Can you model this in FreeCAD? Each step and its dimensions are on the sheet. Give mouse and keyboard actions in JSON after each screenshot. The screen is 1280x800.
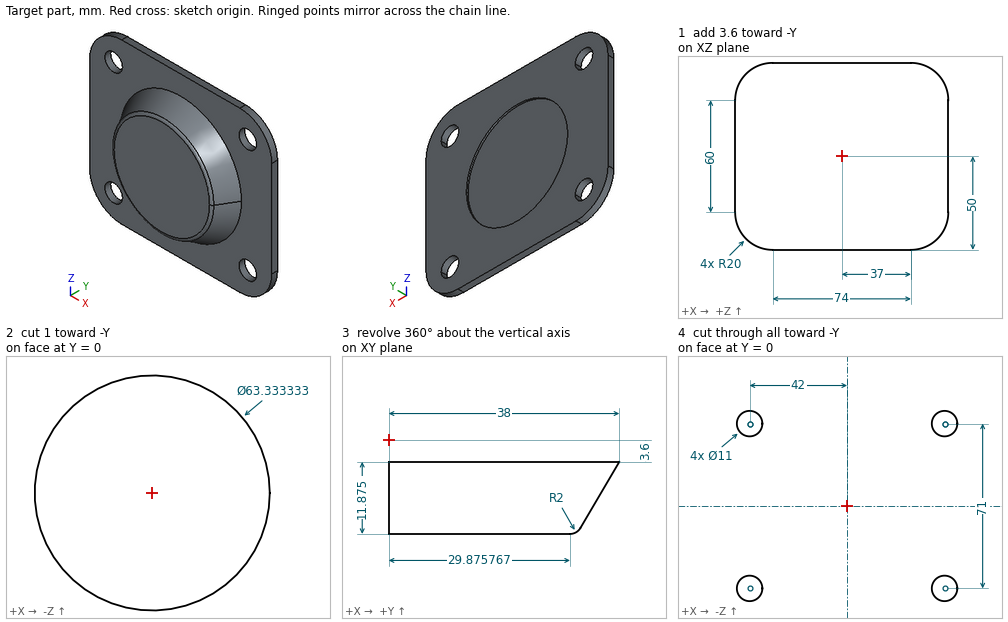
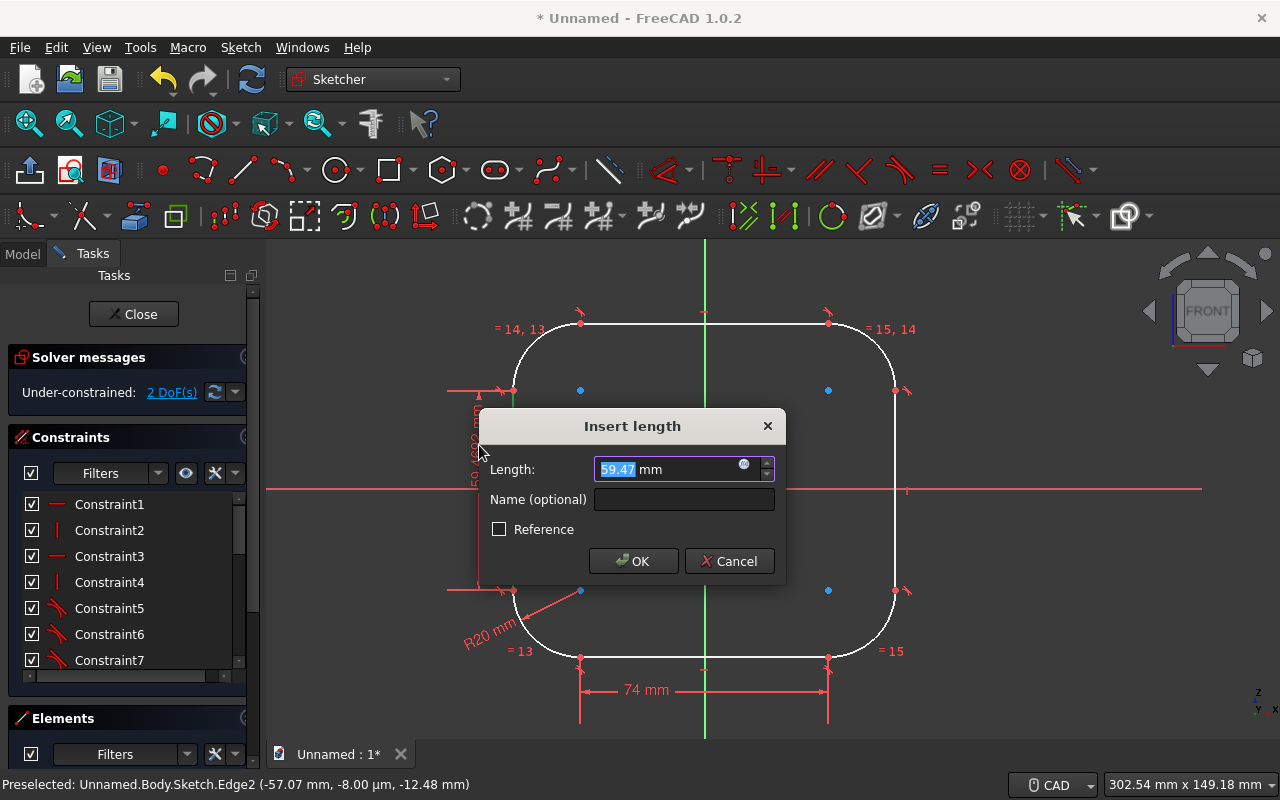
{"action": "type", "text": "60"}
{"action": "key", "text": "Return"}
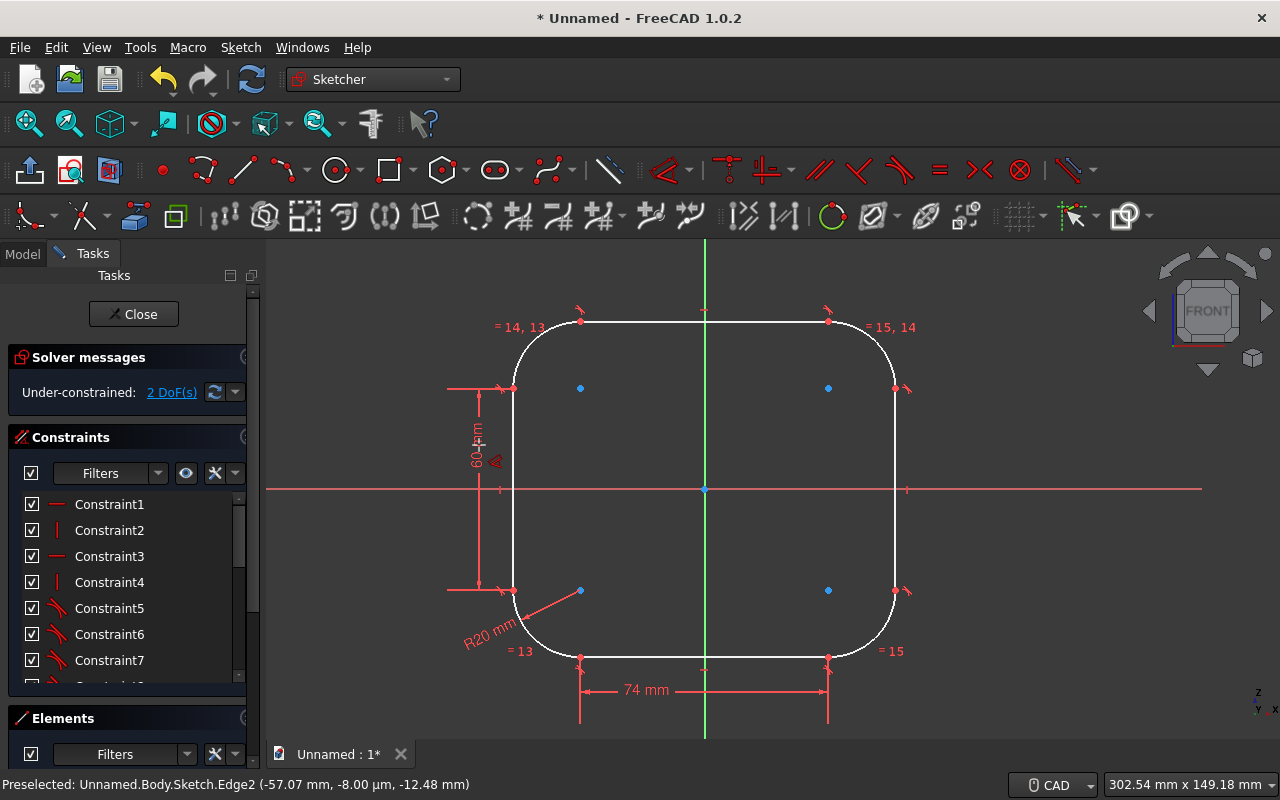
{"action": "left_click", "coordinate": [828, 657]}
{"action": "left_click", "coordinate": [766, 691]}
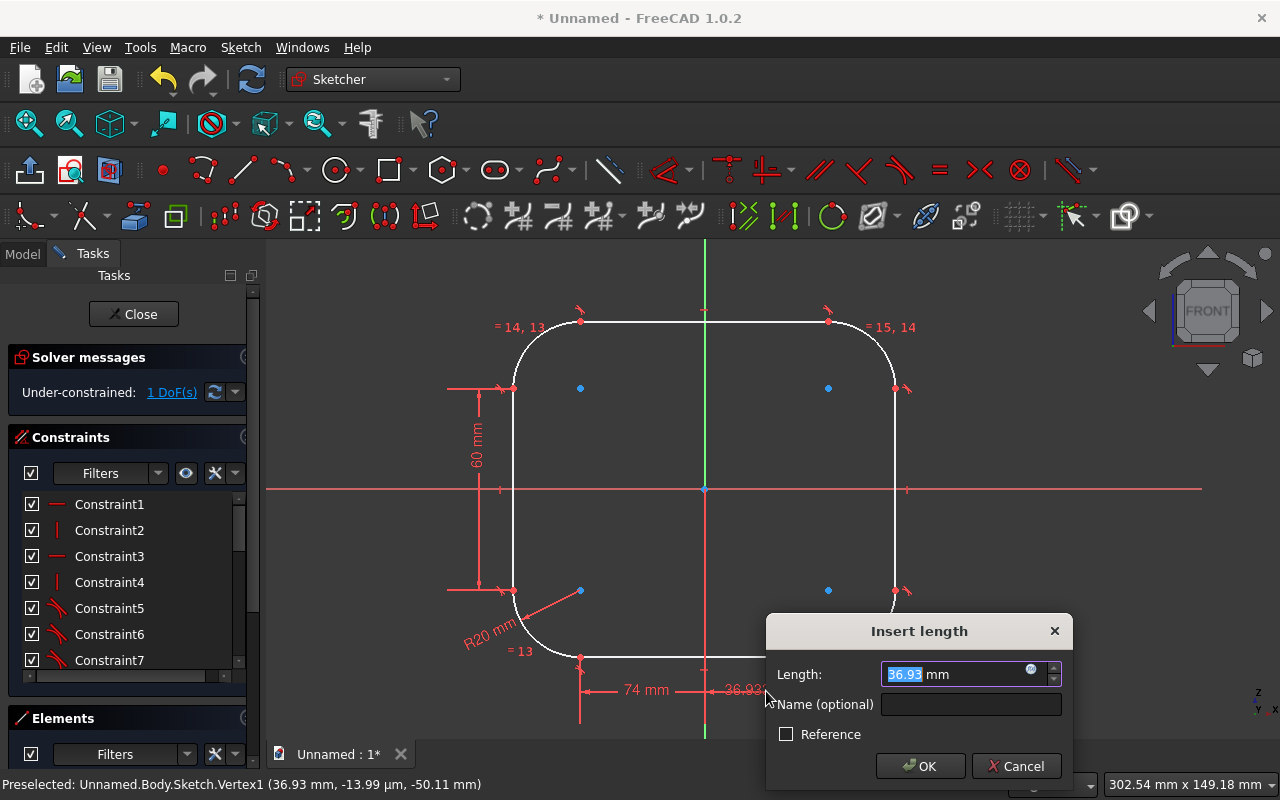
{"action": "type", "text": "37"}
{"action": "key", "text": "Return"}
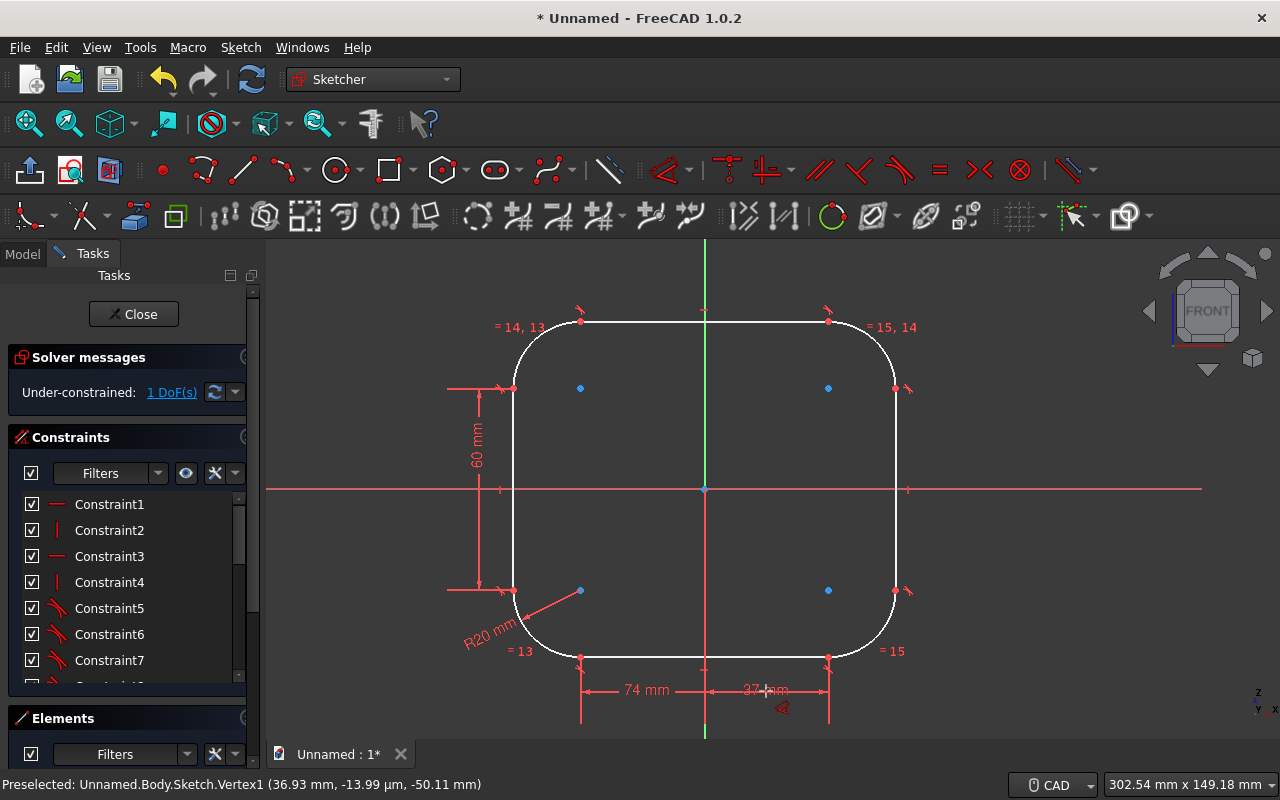
{"action": "left_click", "coordinate": [829, 657]}
{"action": "left_click", "coordinate": [863, 573]}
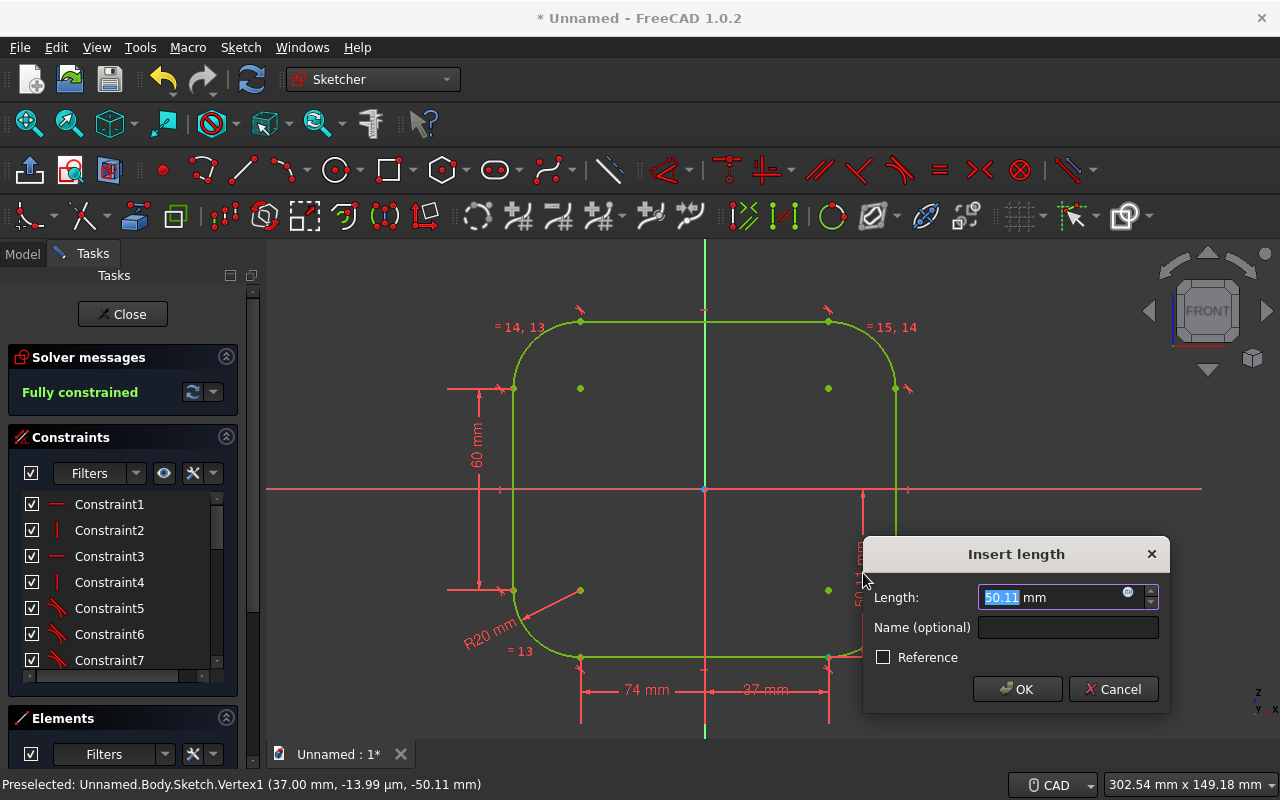
{"action": "type", "text": "50"}
{"action": "key", "text": "Return"}
{"action": "key", "text": "Escape"}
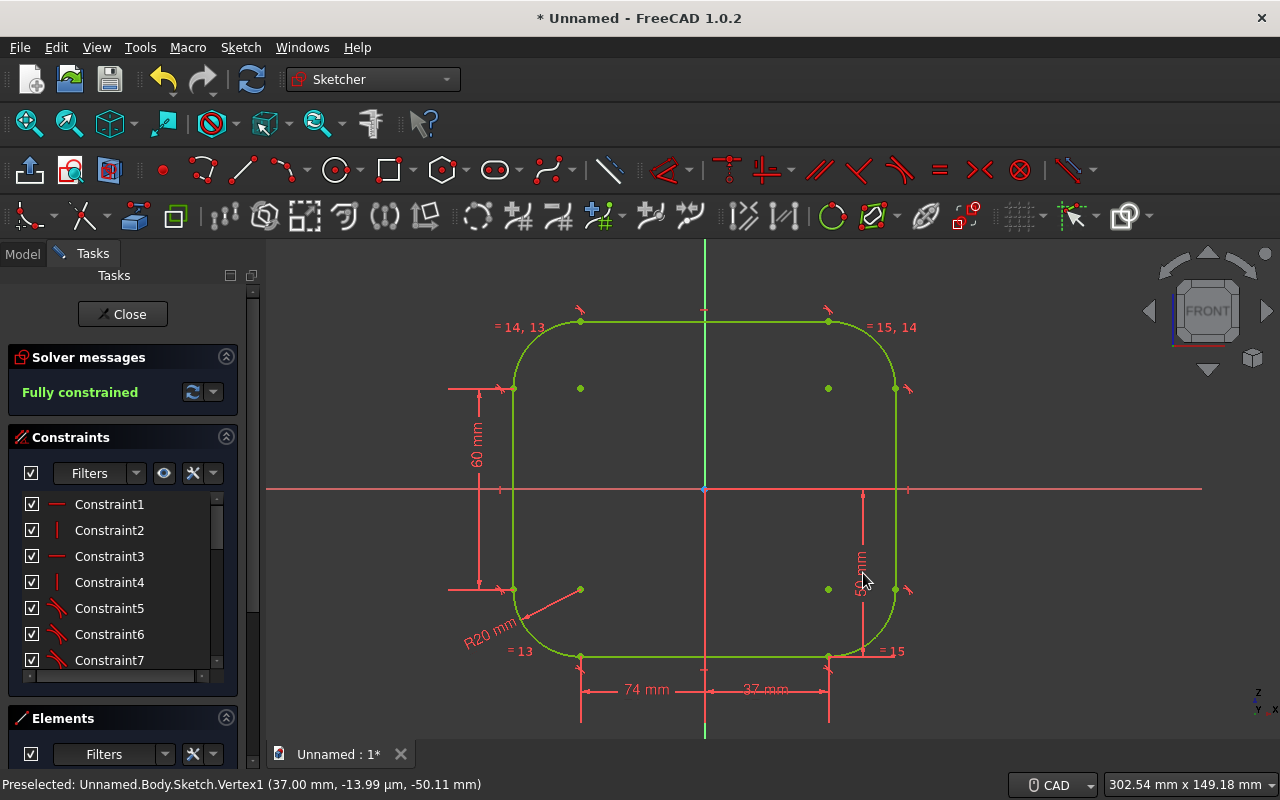
{"action": "left_click", "coordinate": [123, 314]}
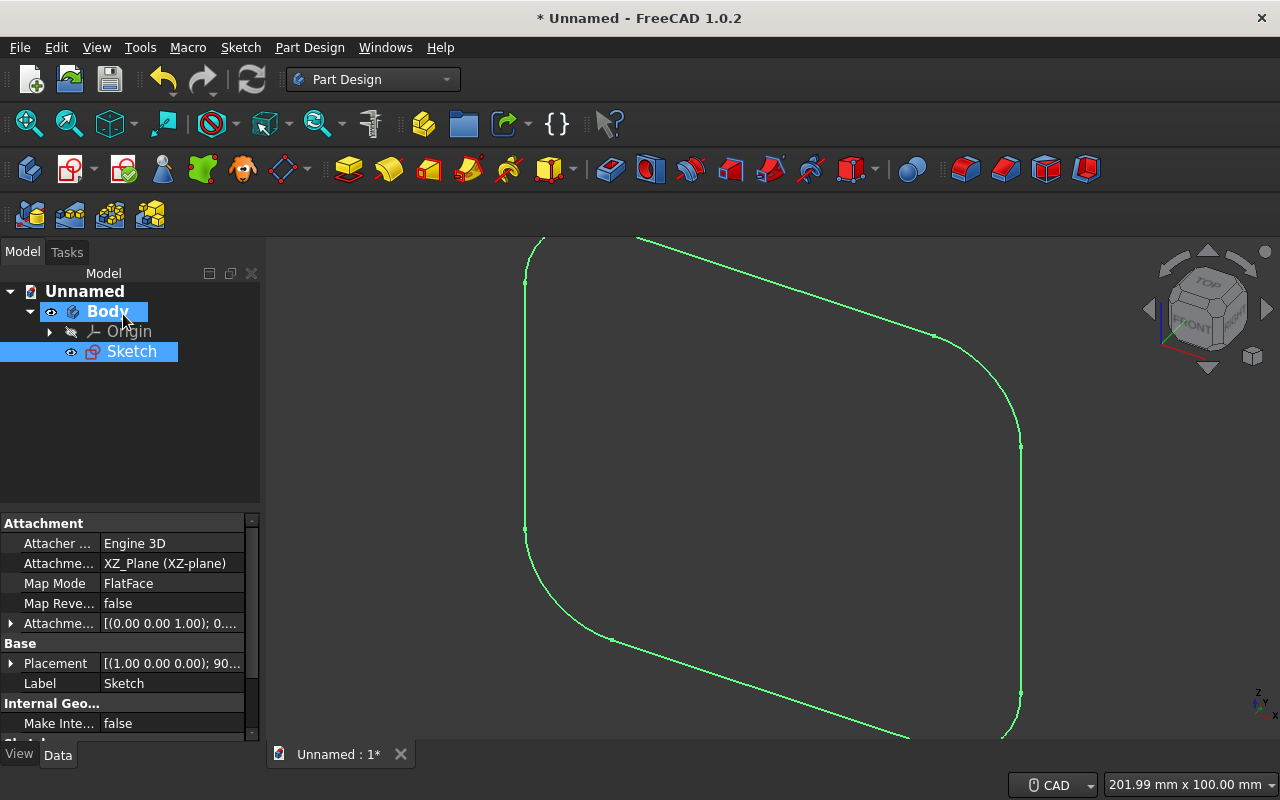
{"action": "left_click", "coordinate": [350, 170]}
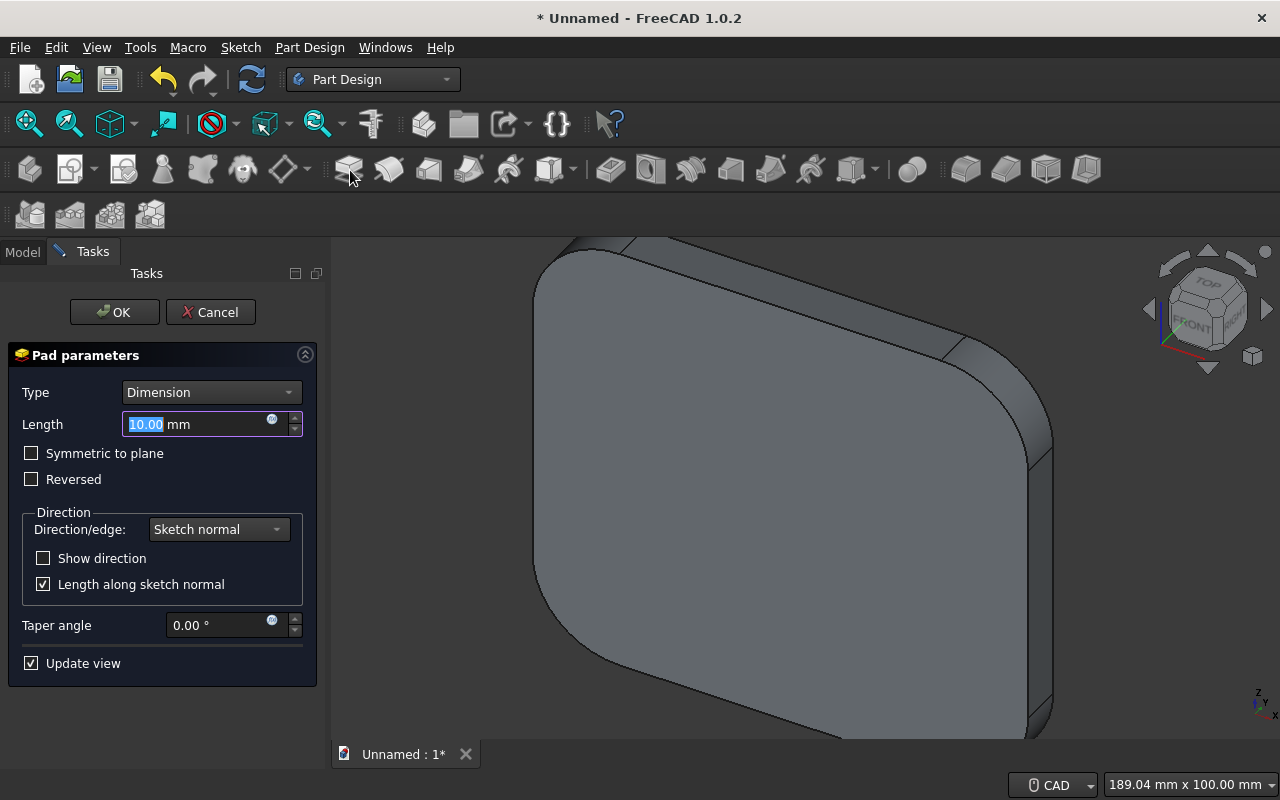
{"action": "type", "text": "3.6"}
{"action": "key", "text": "Tab"}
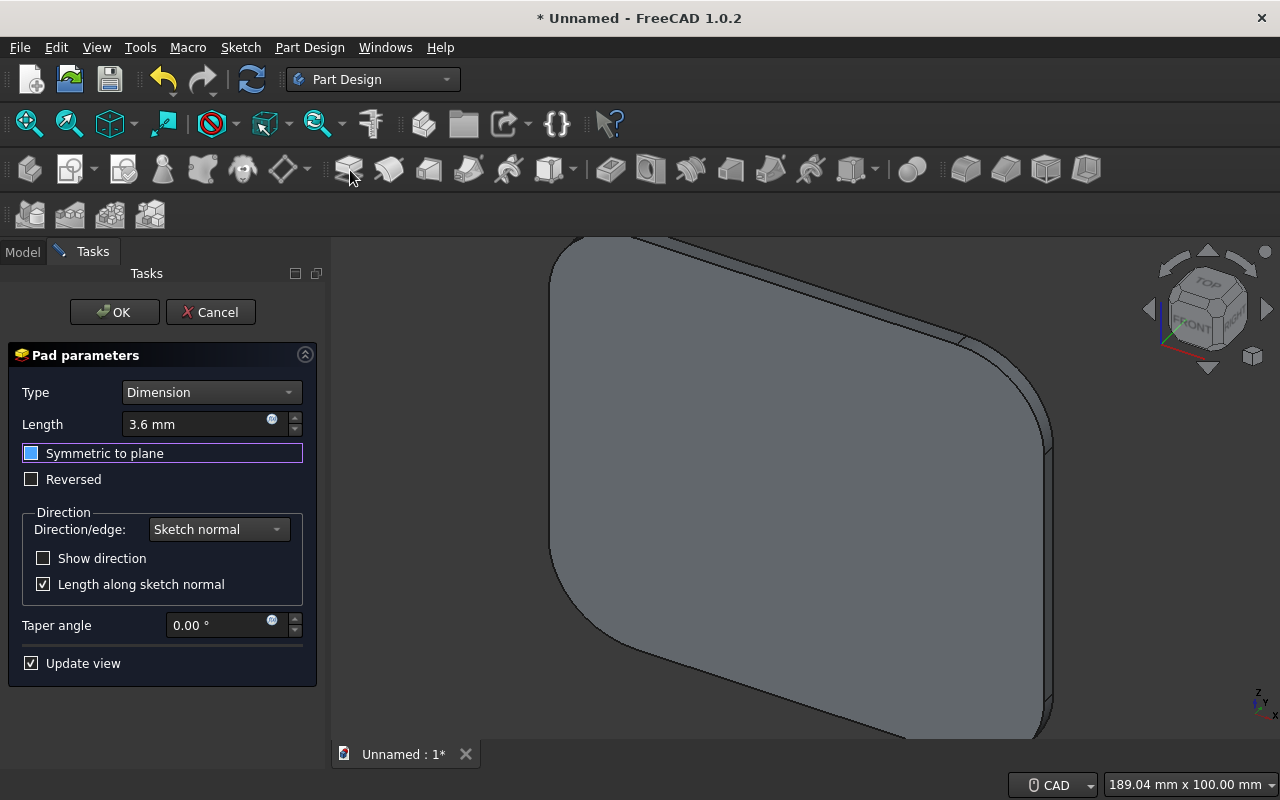
{"action": "left_click", "coordinate": [115, 312]}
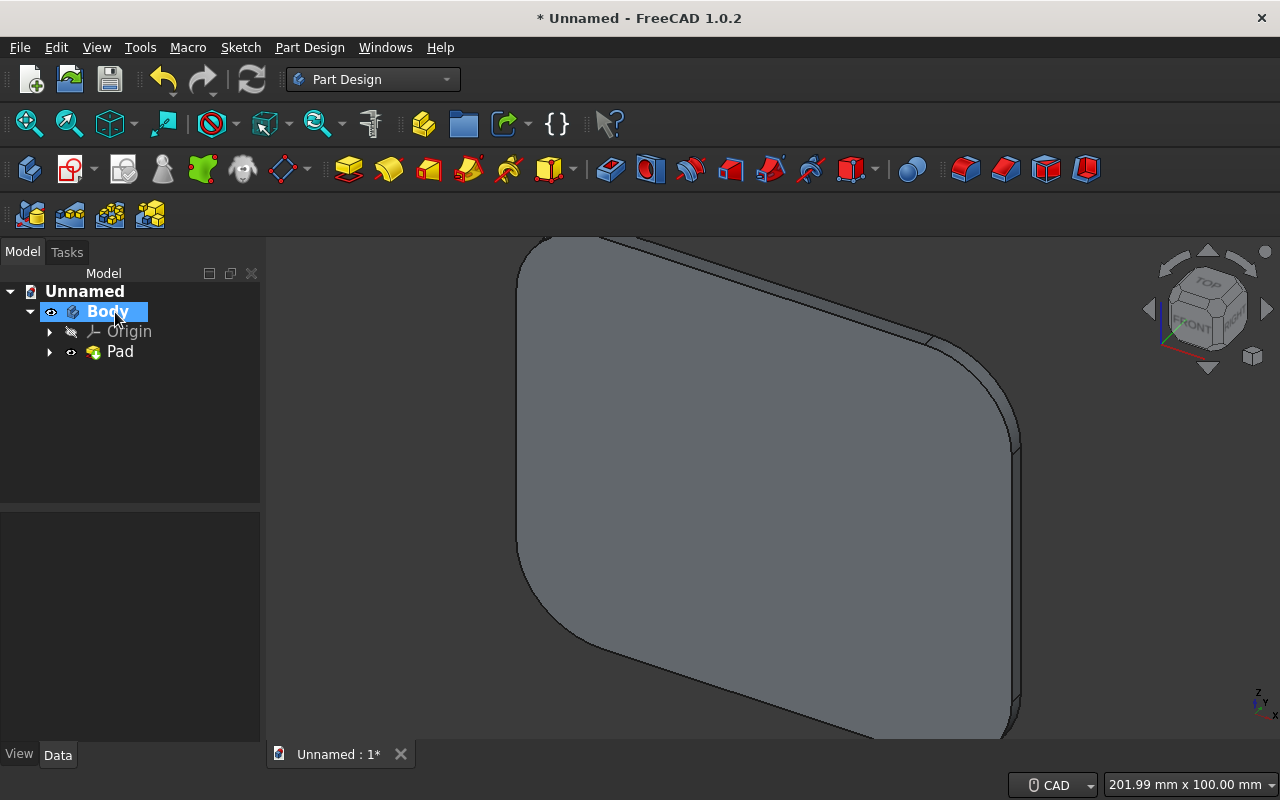
{"action": "left_click", "coordinate": [30, 124]}